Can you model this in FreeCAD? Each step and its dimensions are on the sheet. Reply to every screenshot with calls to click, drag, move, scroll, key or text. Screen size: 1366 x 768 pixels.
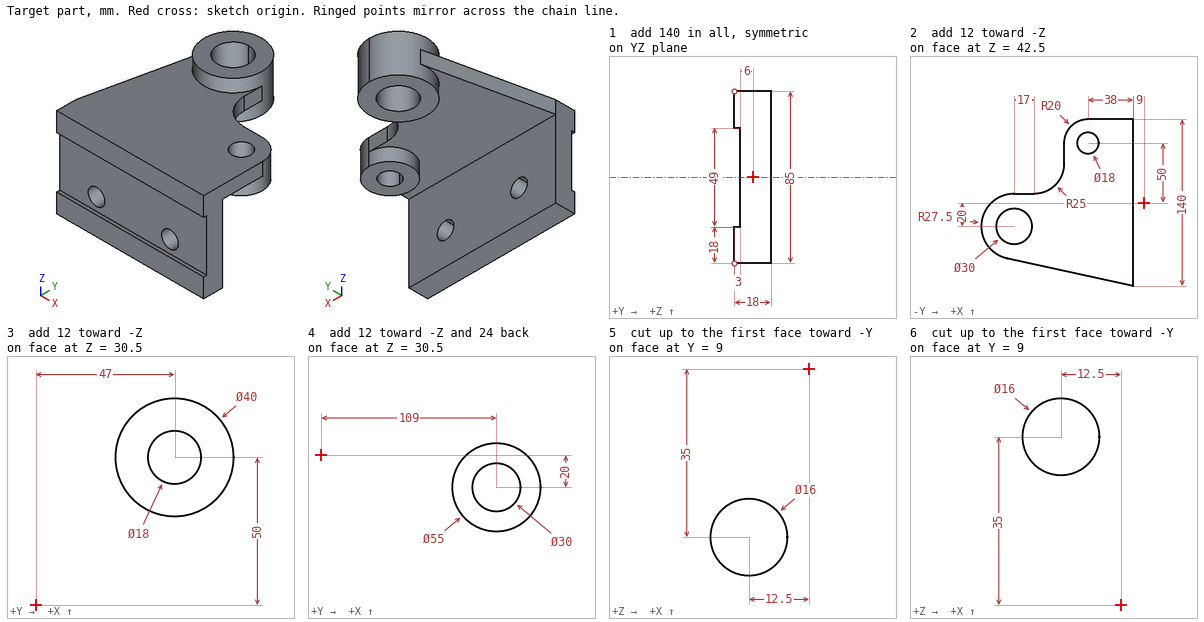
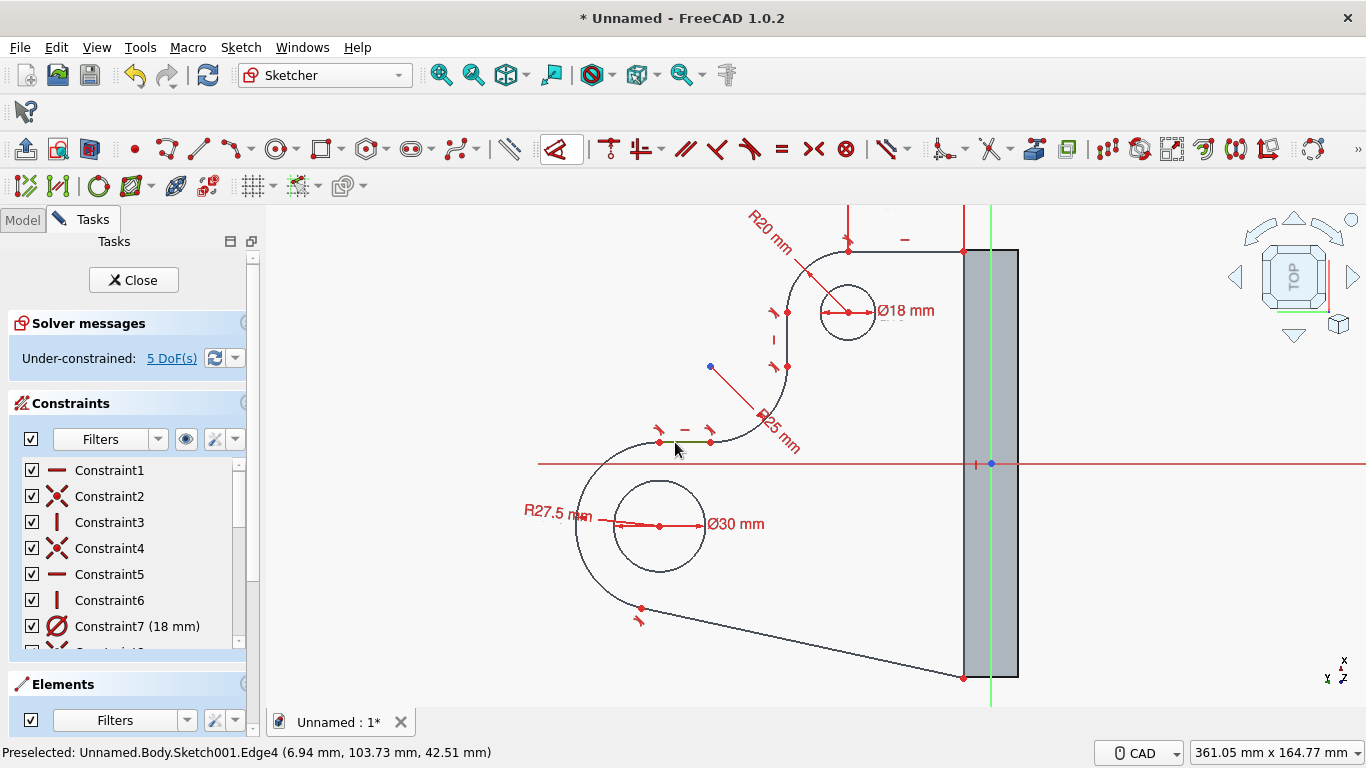
key(l)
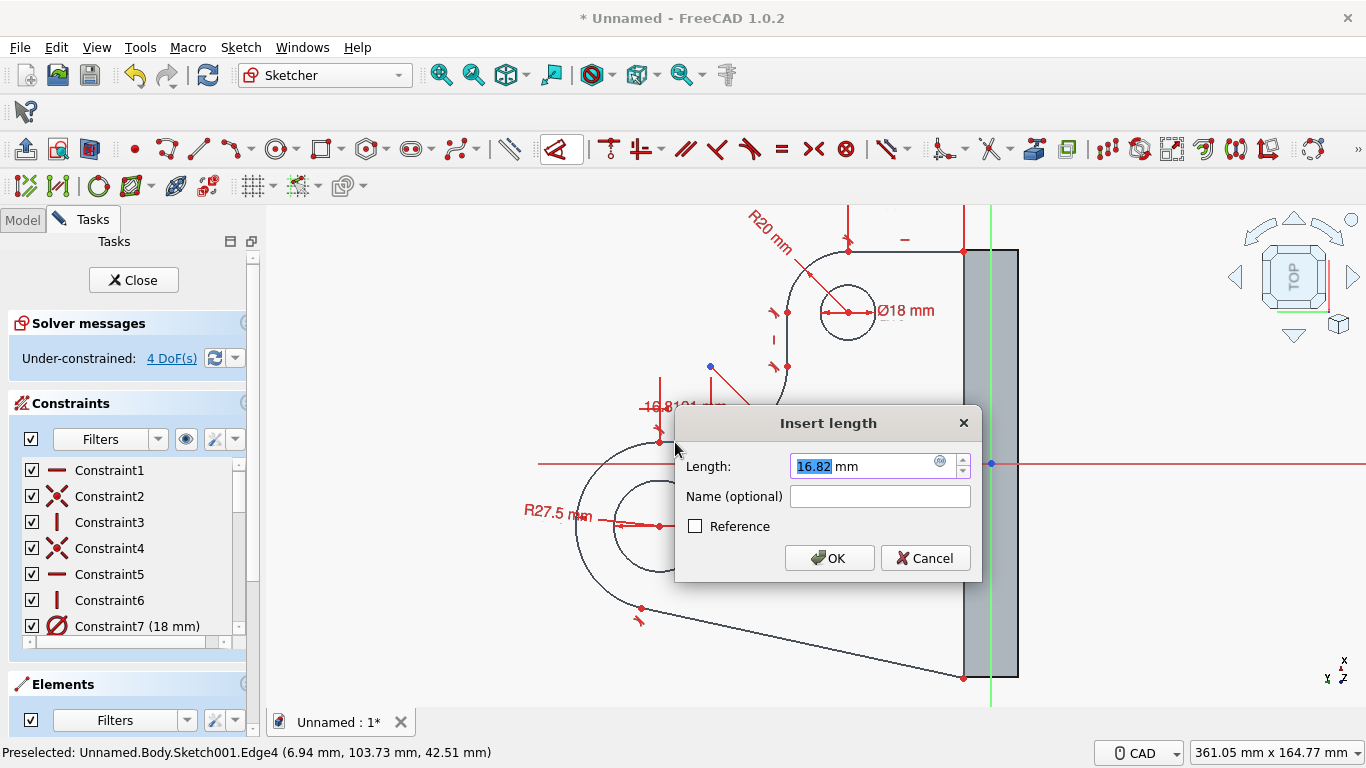
text(17)
key(Return)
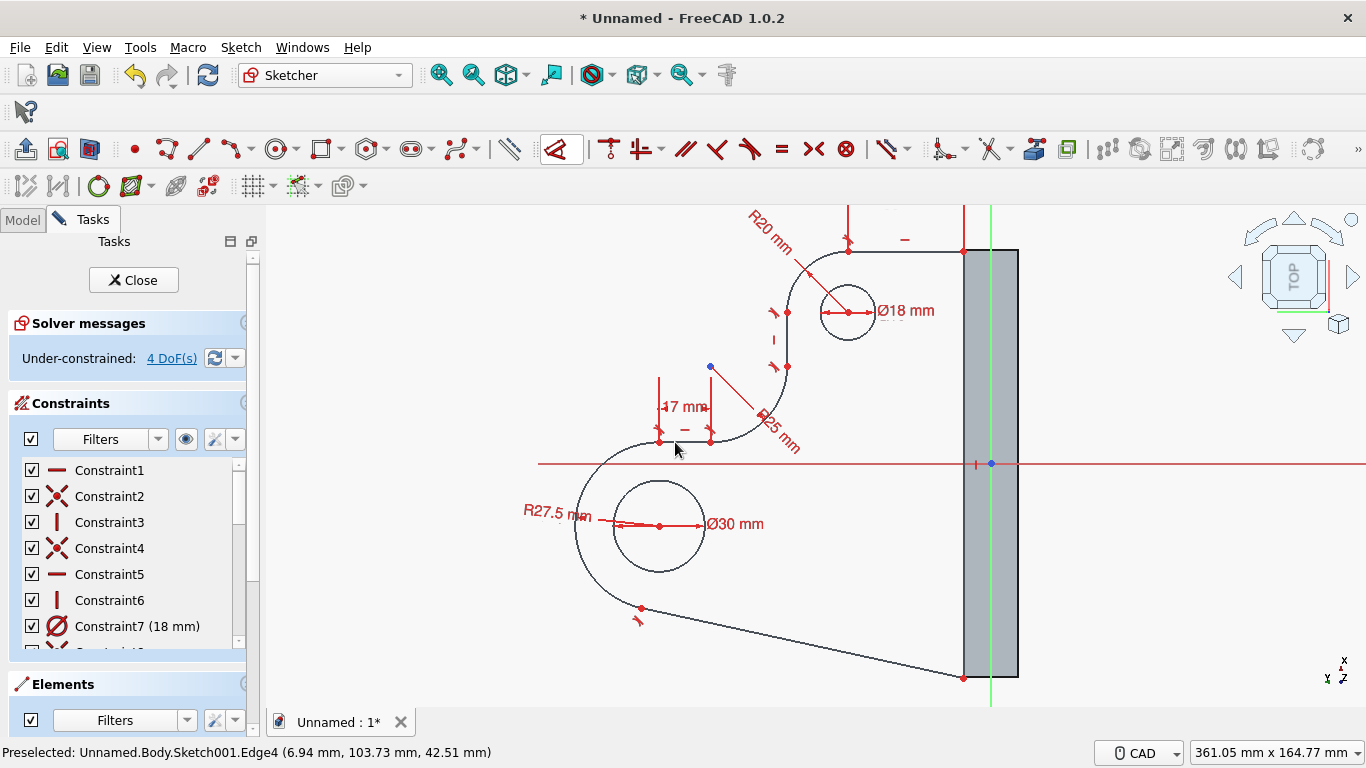
scroll(964, 252, up, 2)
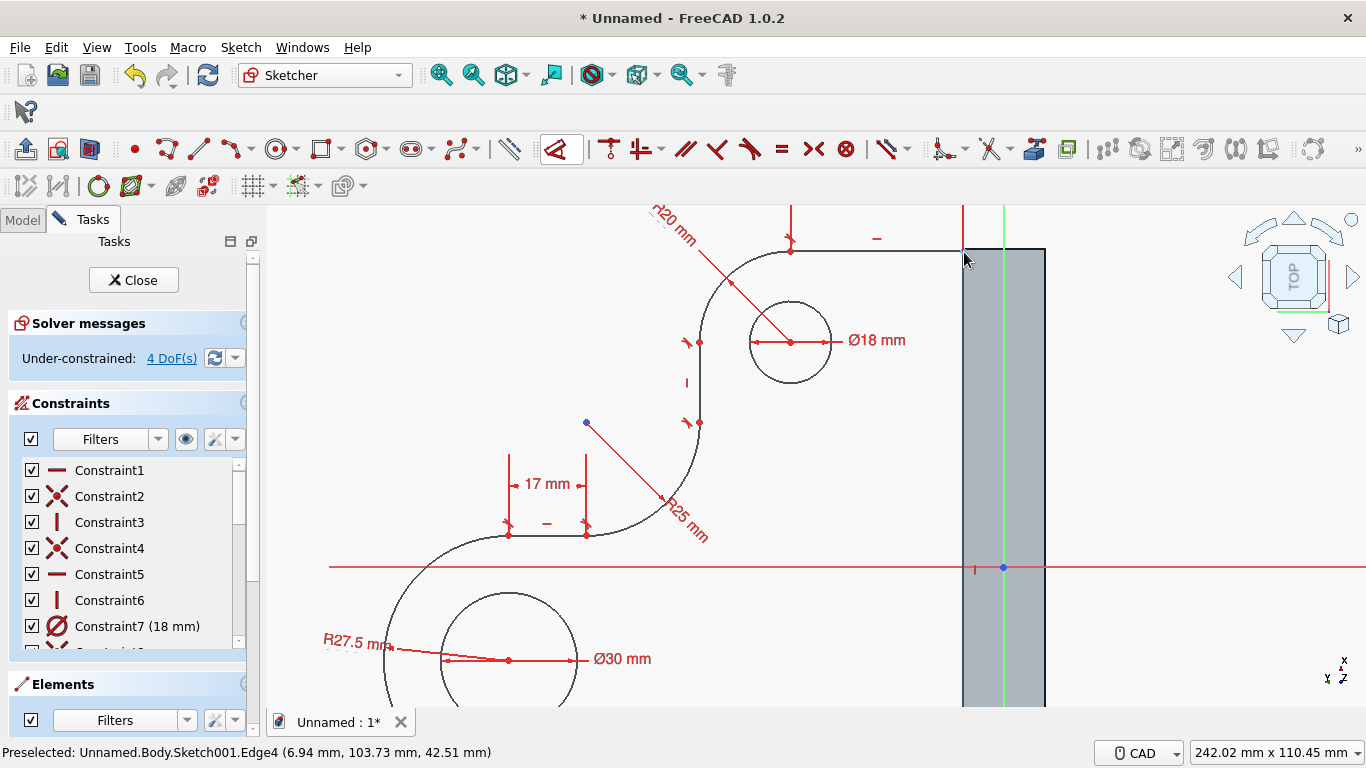
click(963, 251)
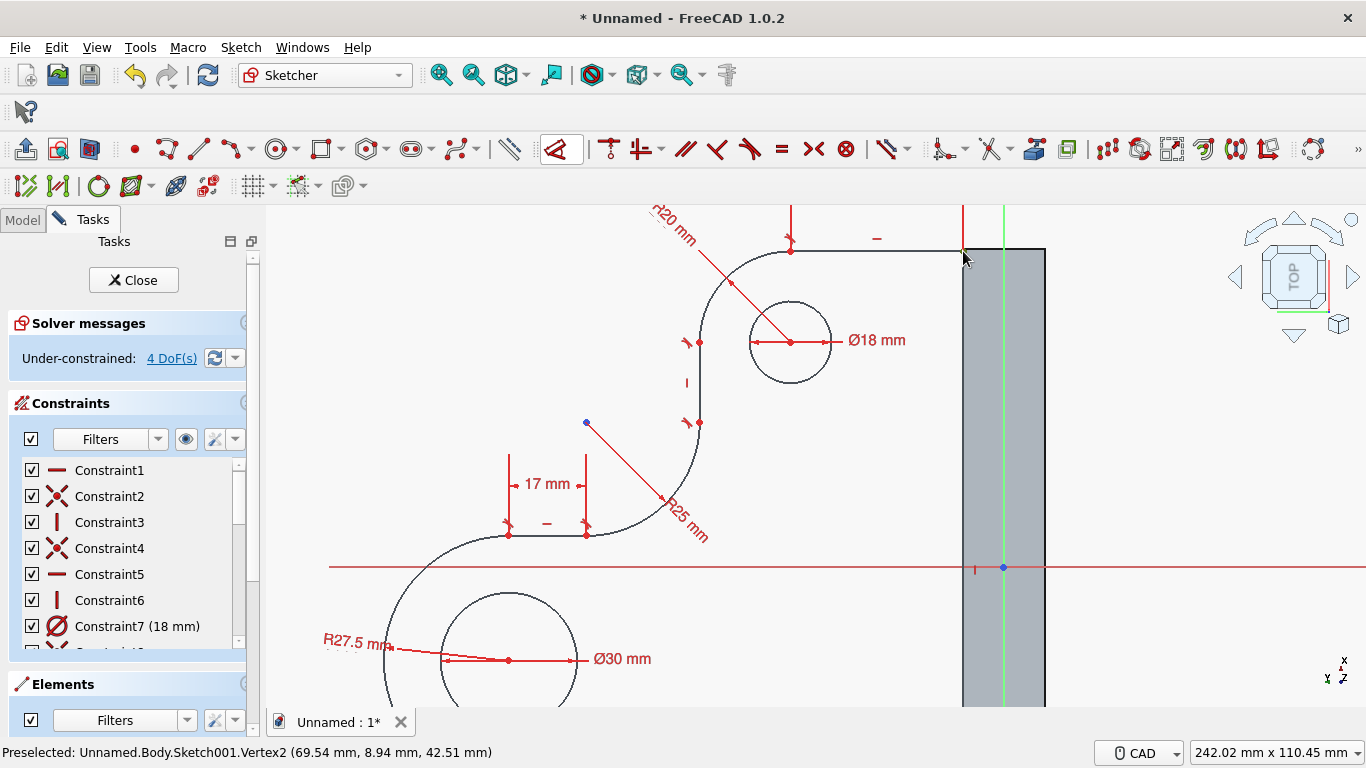
key(l)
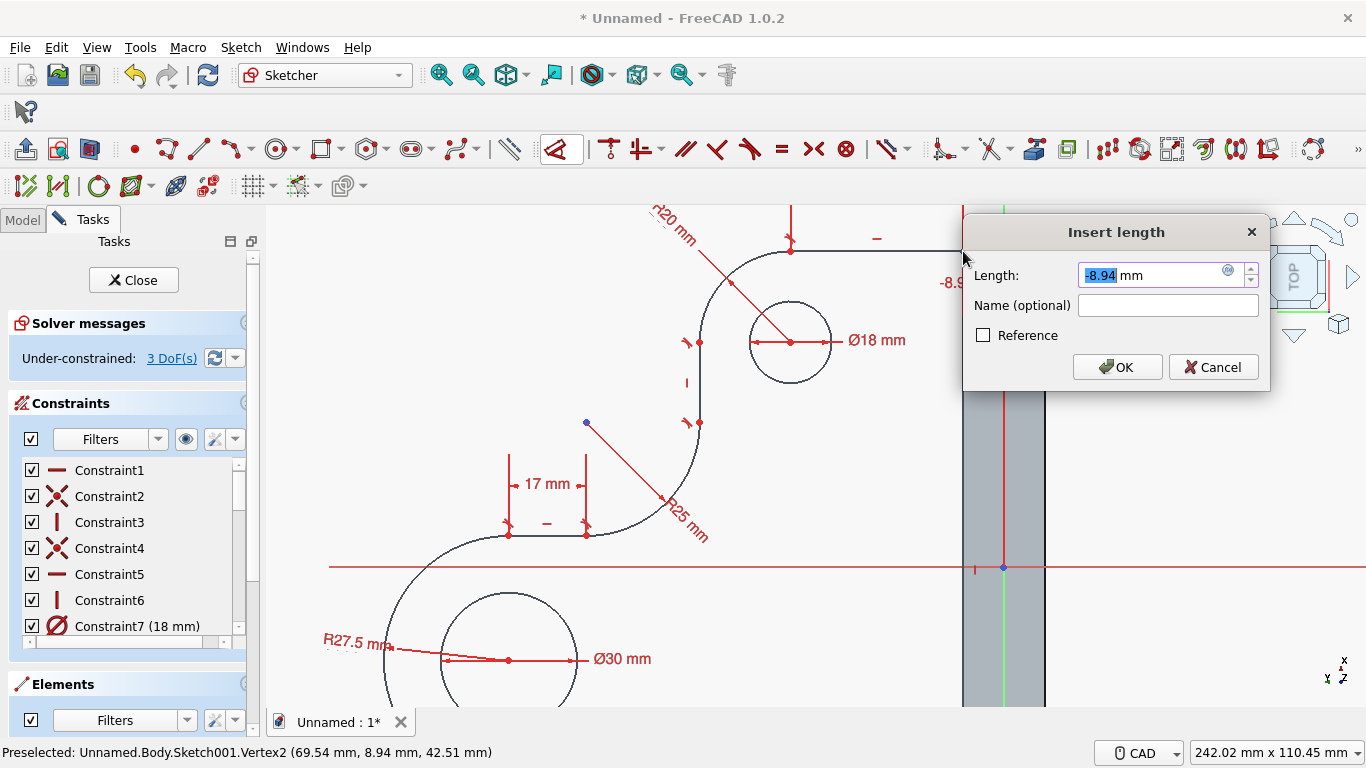
text(-9)
key(Return)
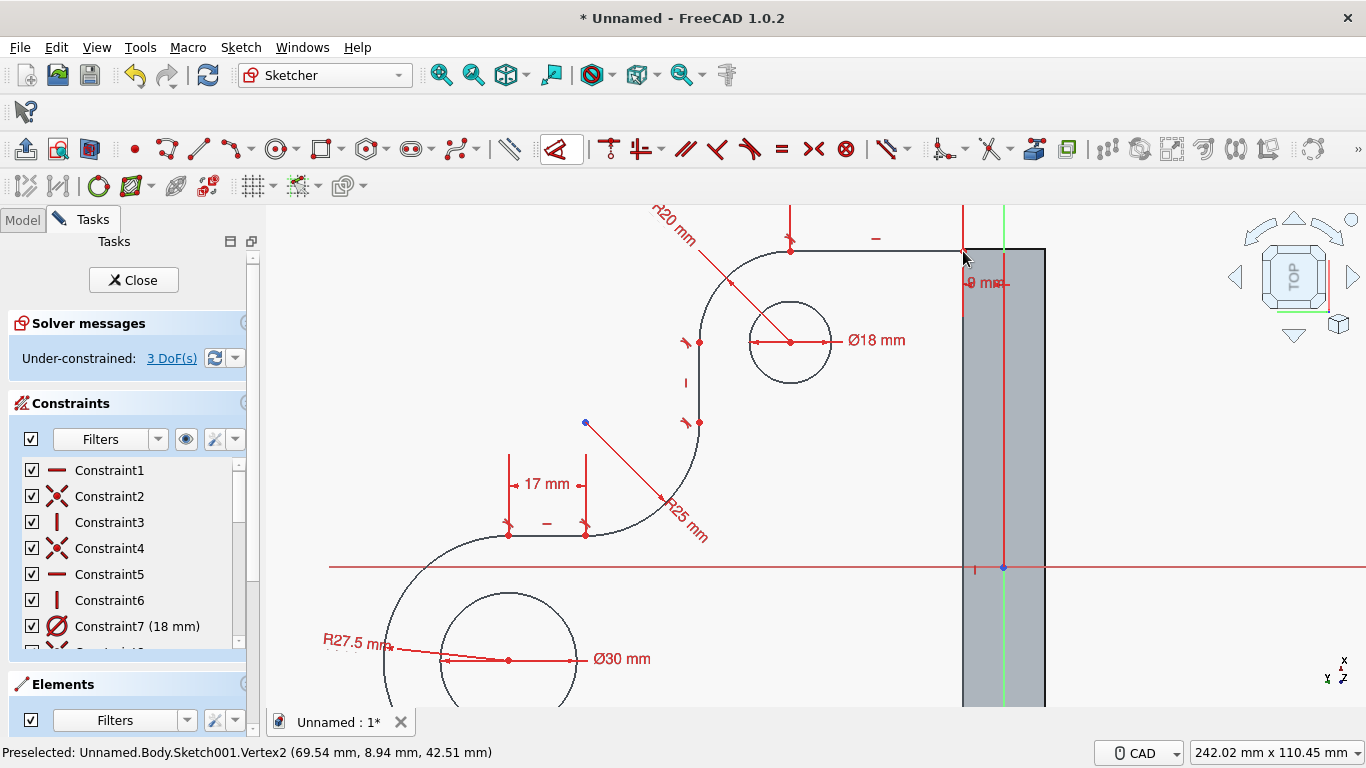
click(790, 342)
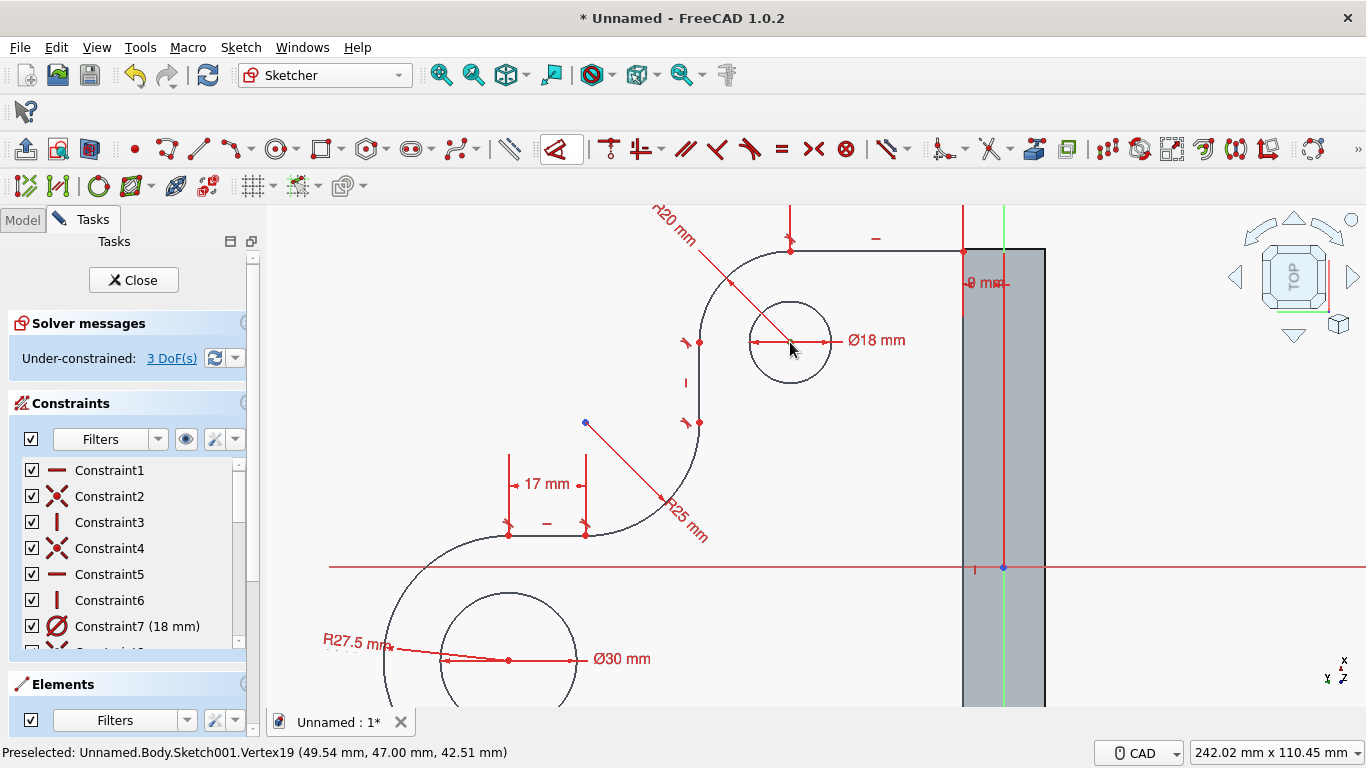
key(i)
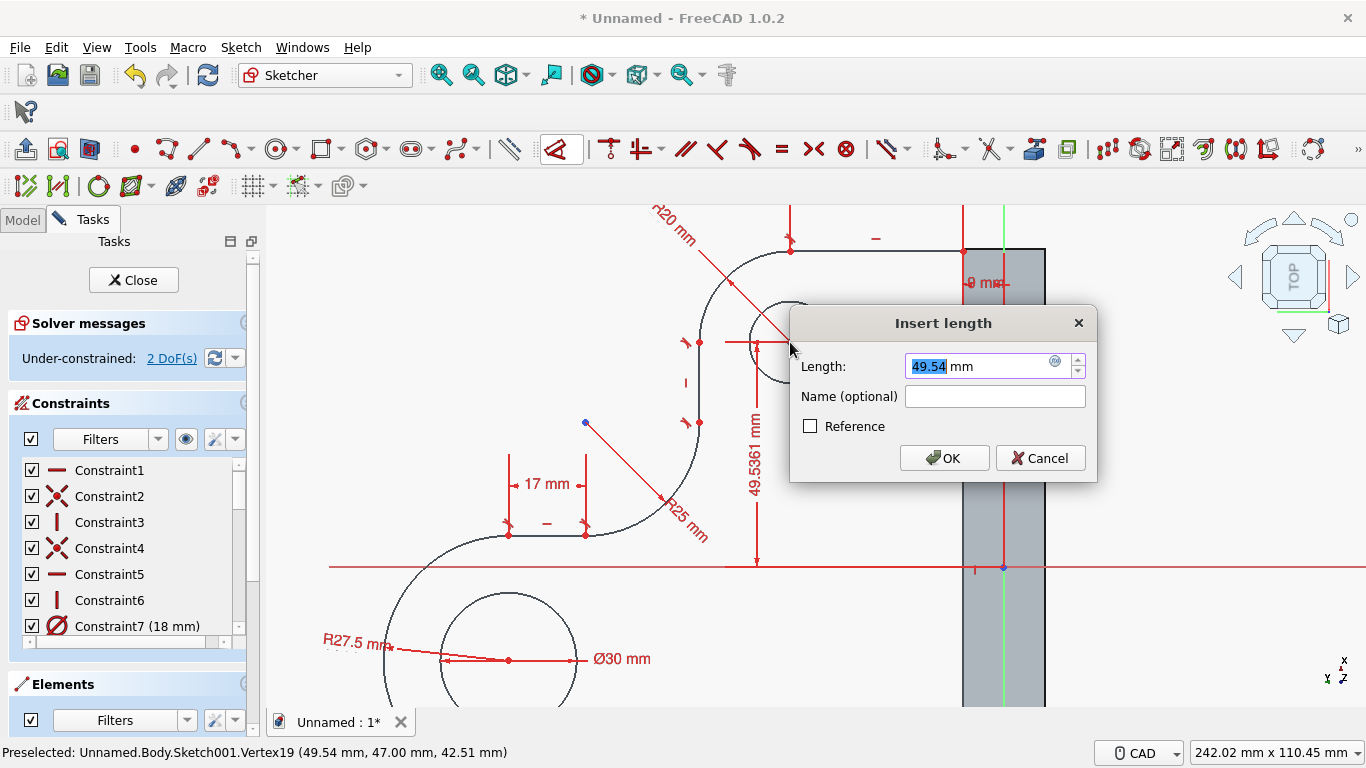
text(50)
key(Return)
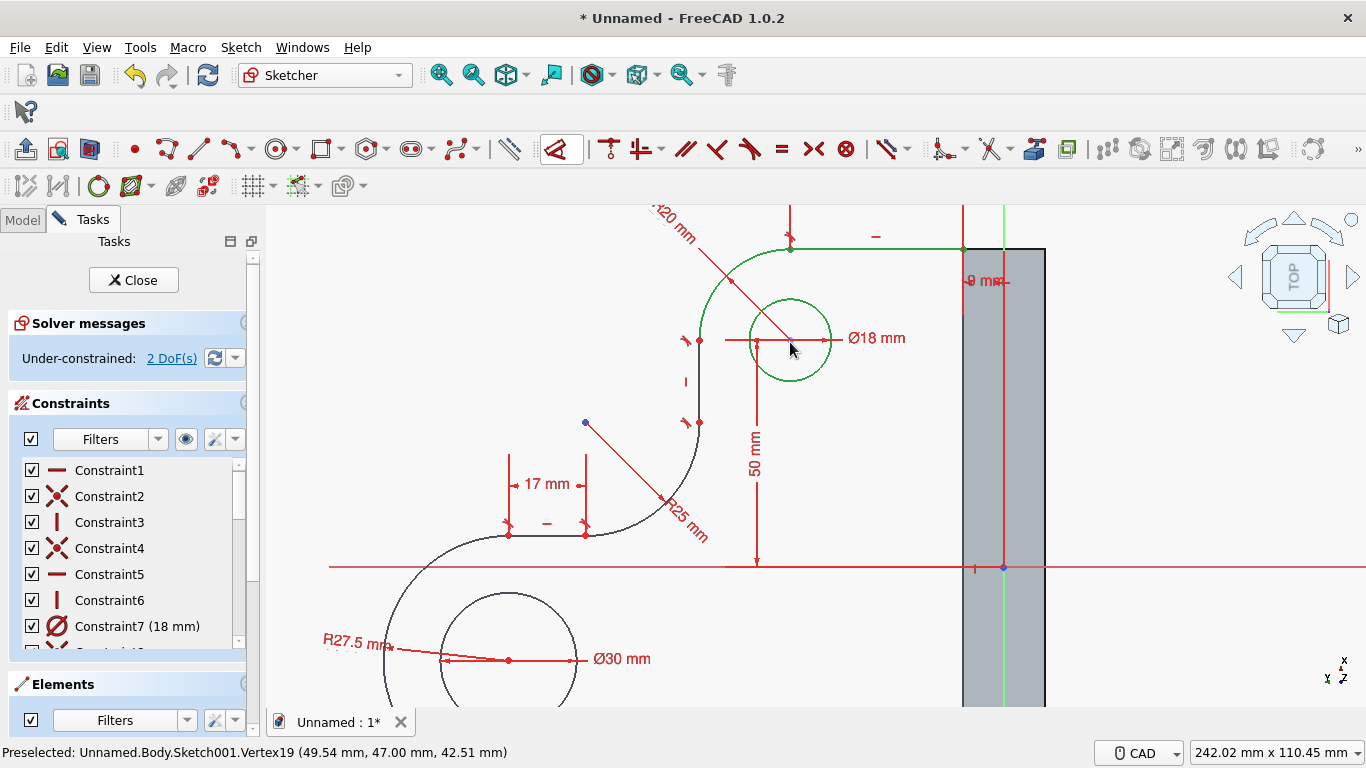
click(509, 661)